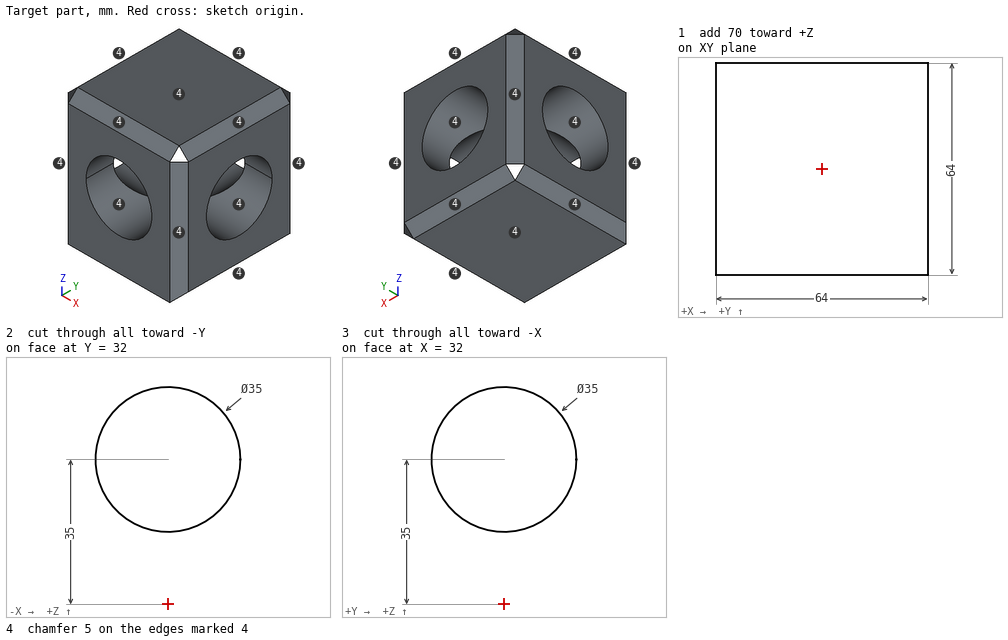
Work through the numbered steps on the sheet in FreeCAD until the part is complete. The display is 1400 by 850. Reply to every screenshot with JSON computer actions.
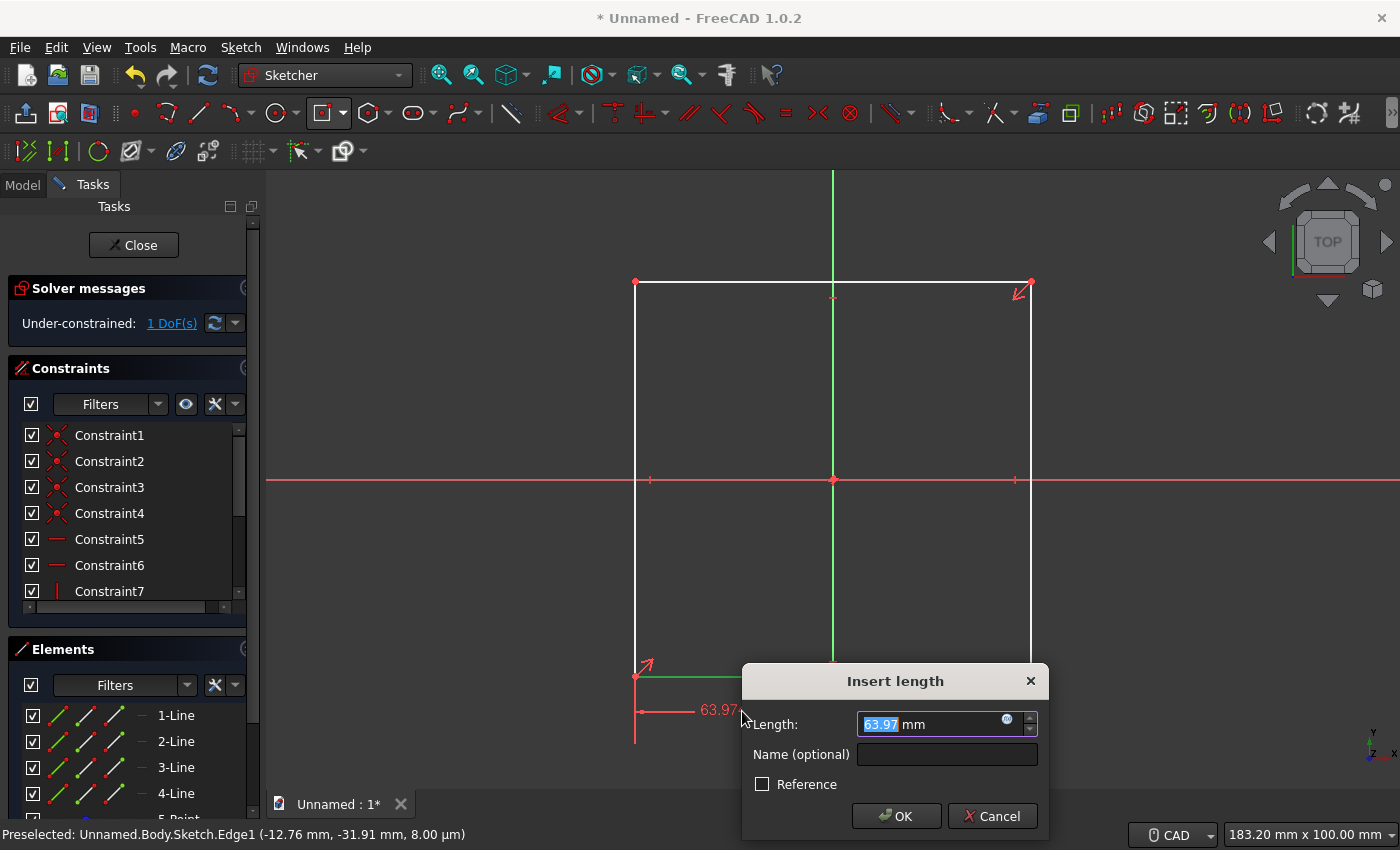
{"action": "type", "text": "64"}
{"action": "key", "text": "Return"}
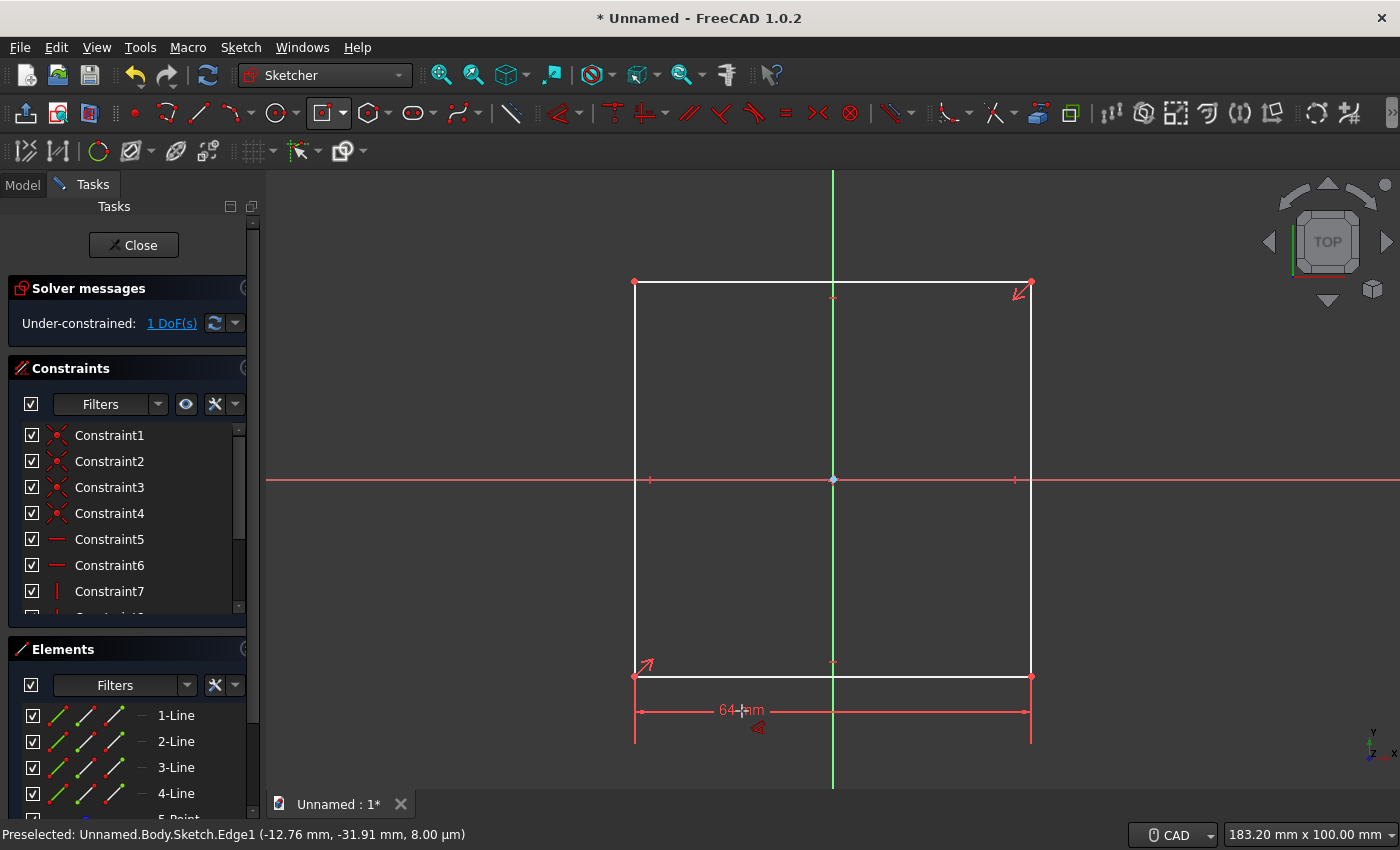
{"action": "left_click", "coordinate": [1031, 559]}
{"action": "left_click", "coordinate": [1065, 389]}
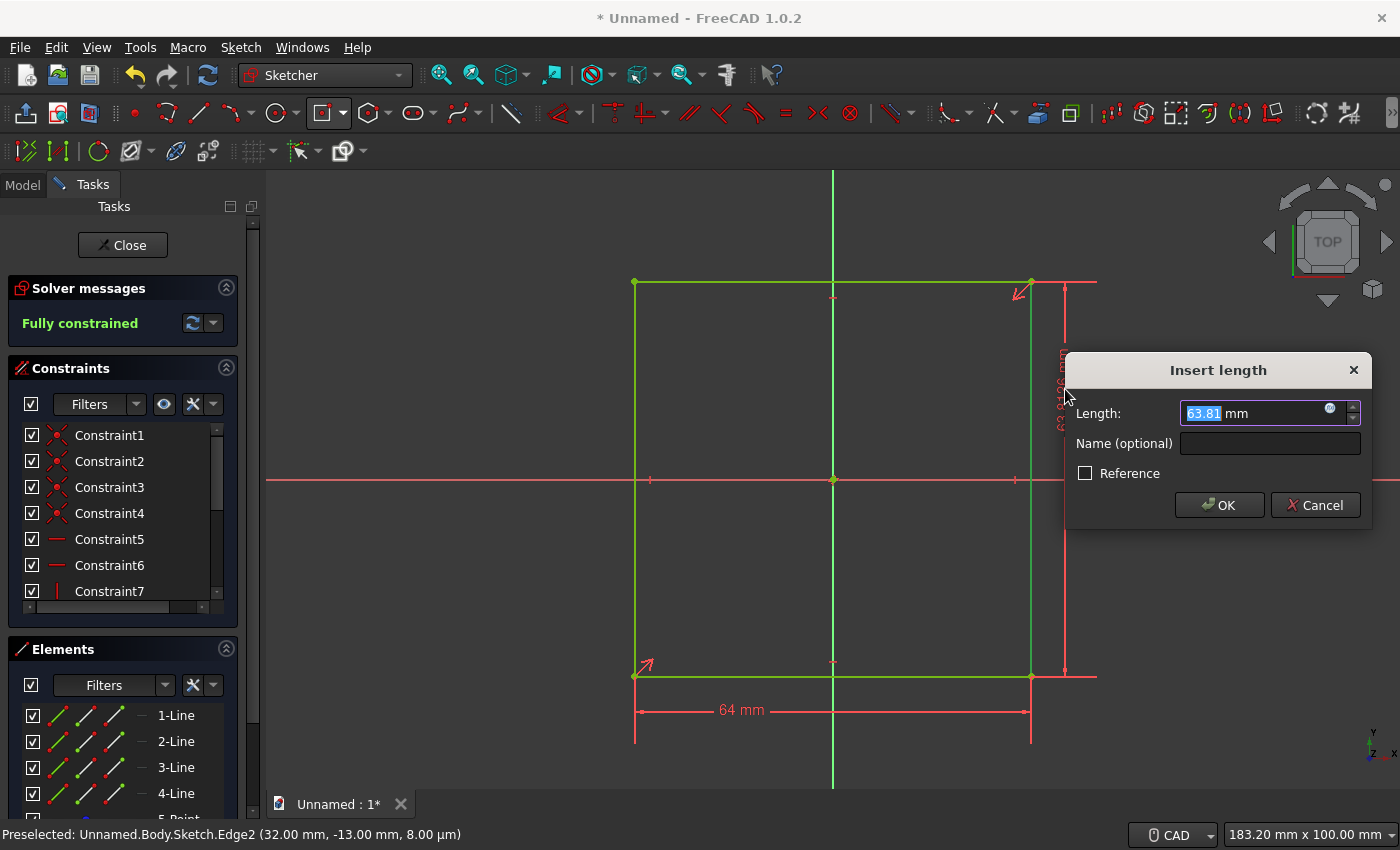
{"action": "type", "text": "64"}
{"action": "key", "text": "Return"}
{"action": "key", "text": "Escape"}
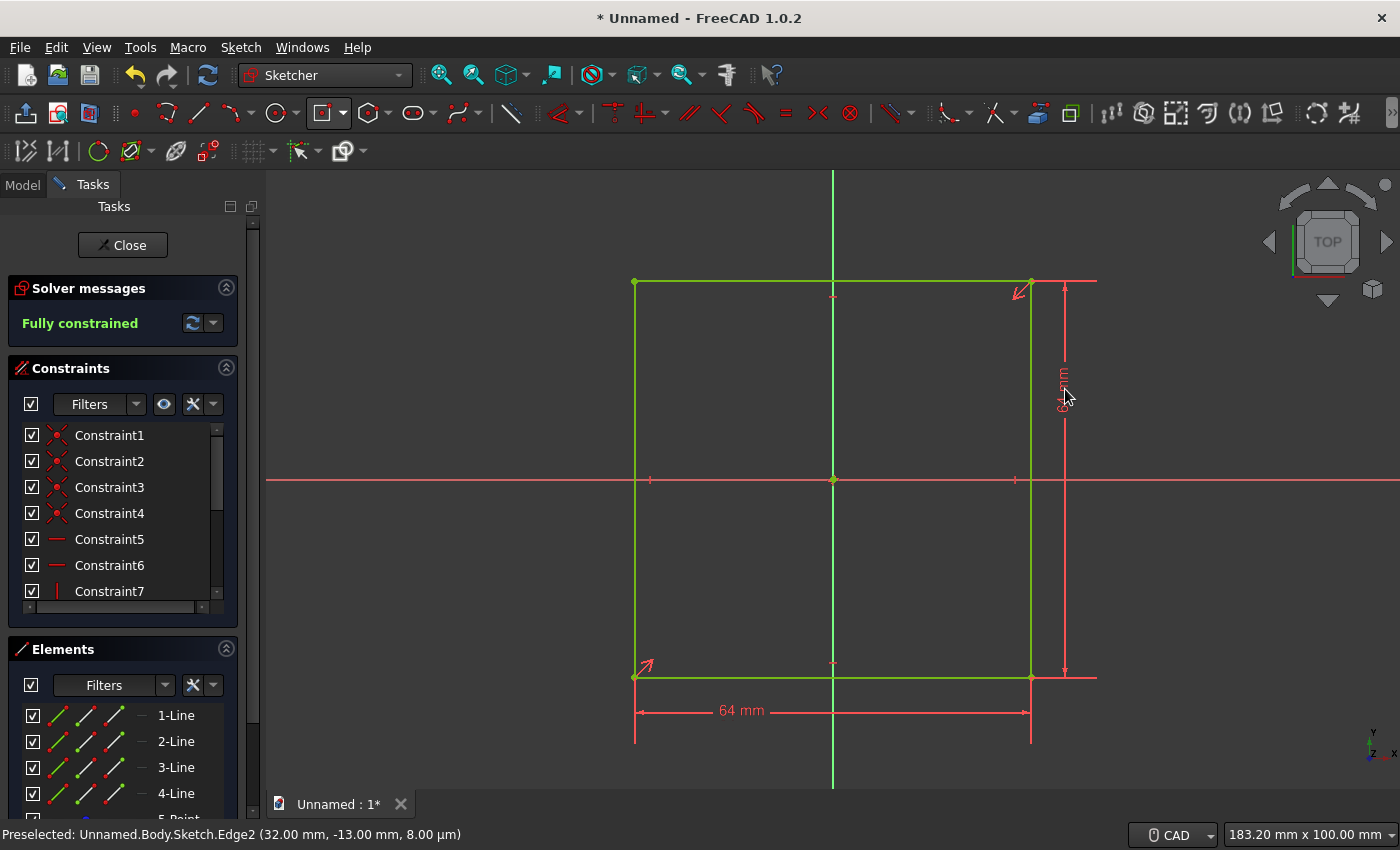
{"action": "left_click", "coordinate": [123, 245]}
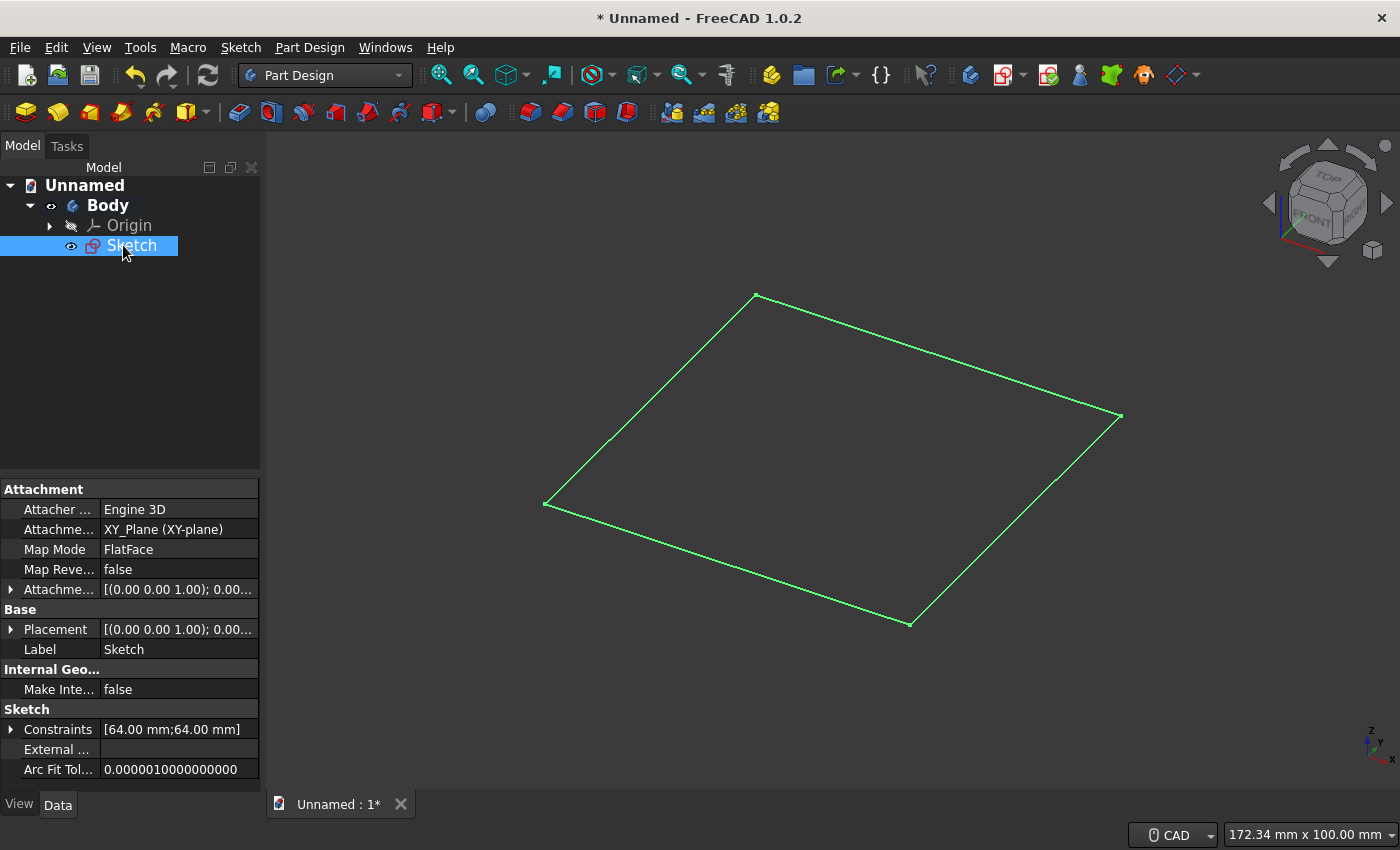
{"action": "left_click", "coordinate": [26, 112]}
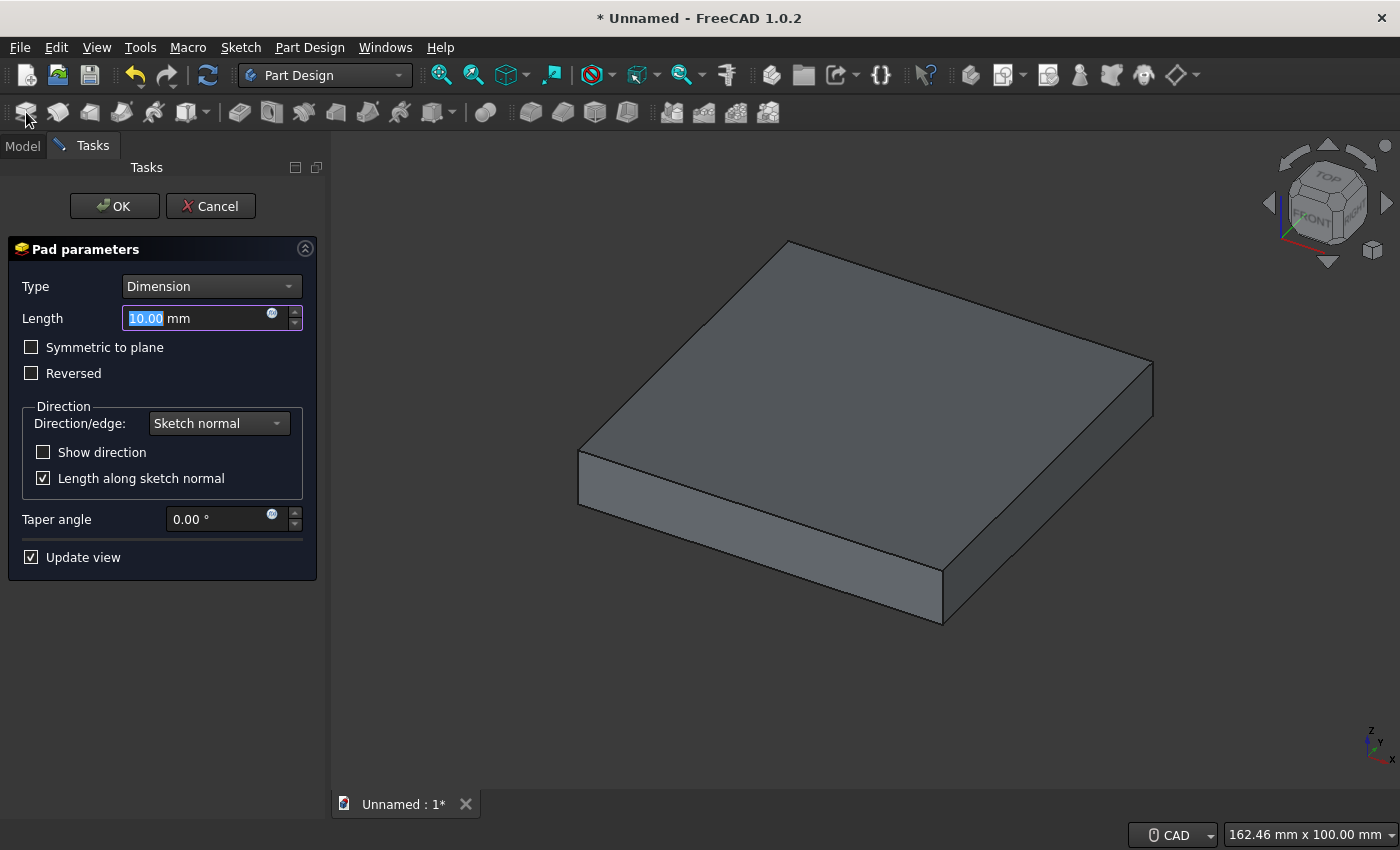
{"action": "type", "text": "70"}
{"action": "key", "text": "Tab"}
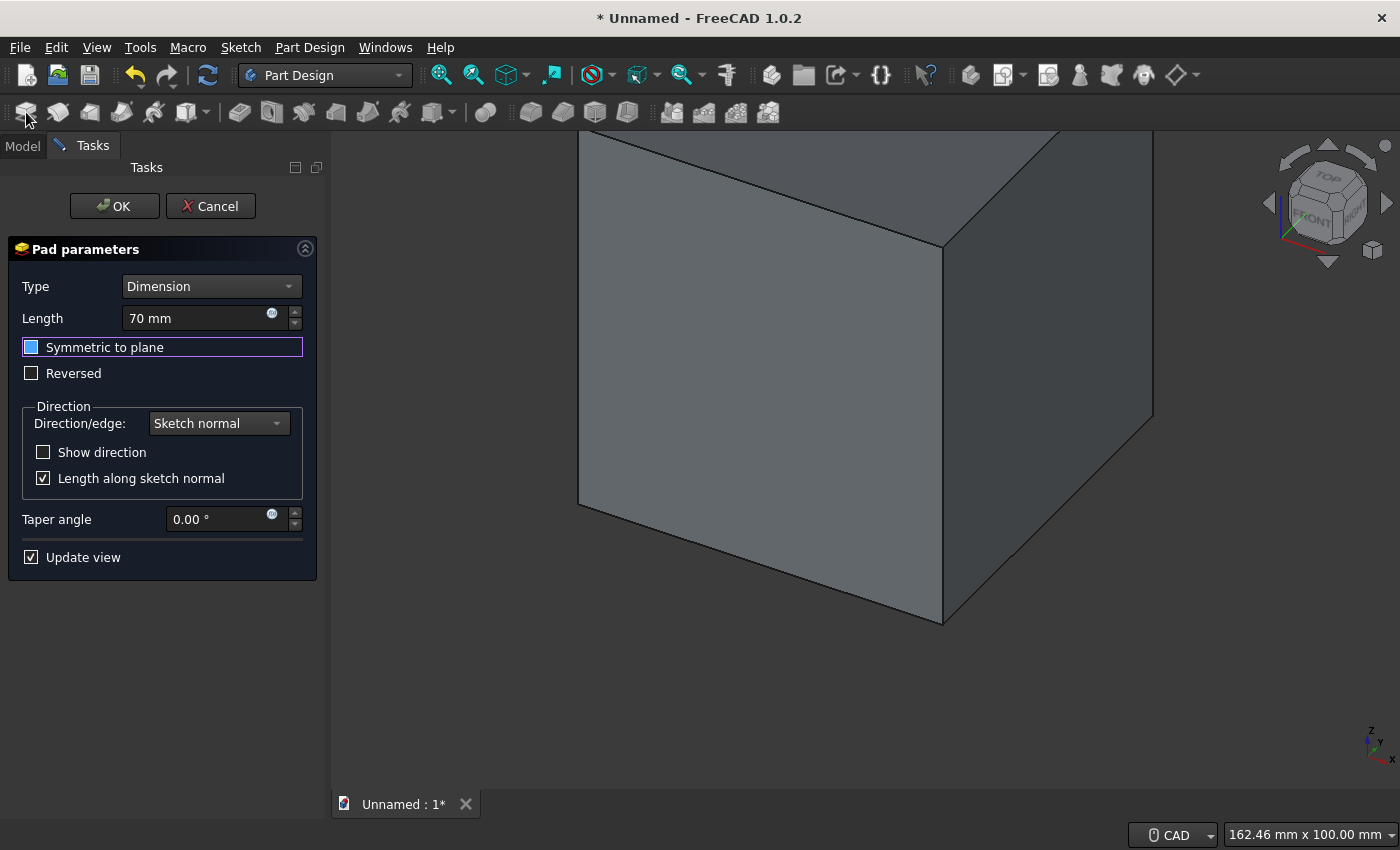
{"action": "left_click", "coordinate": [115, 206]}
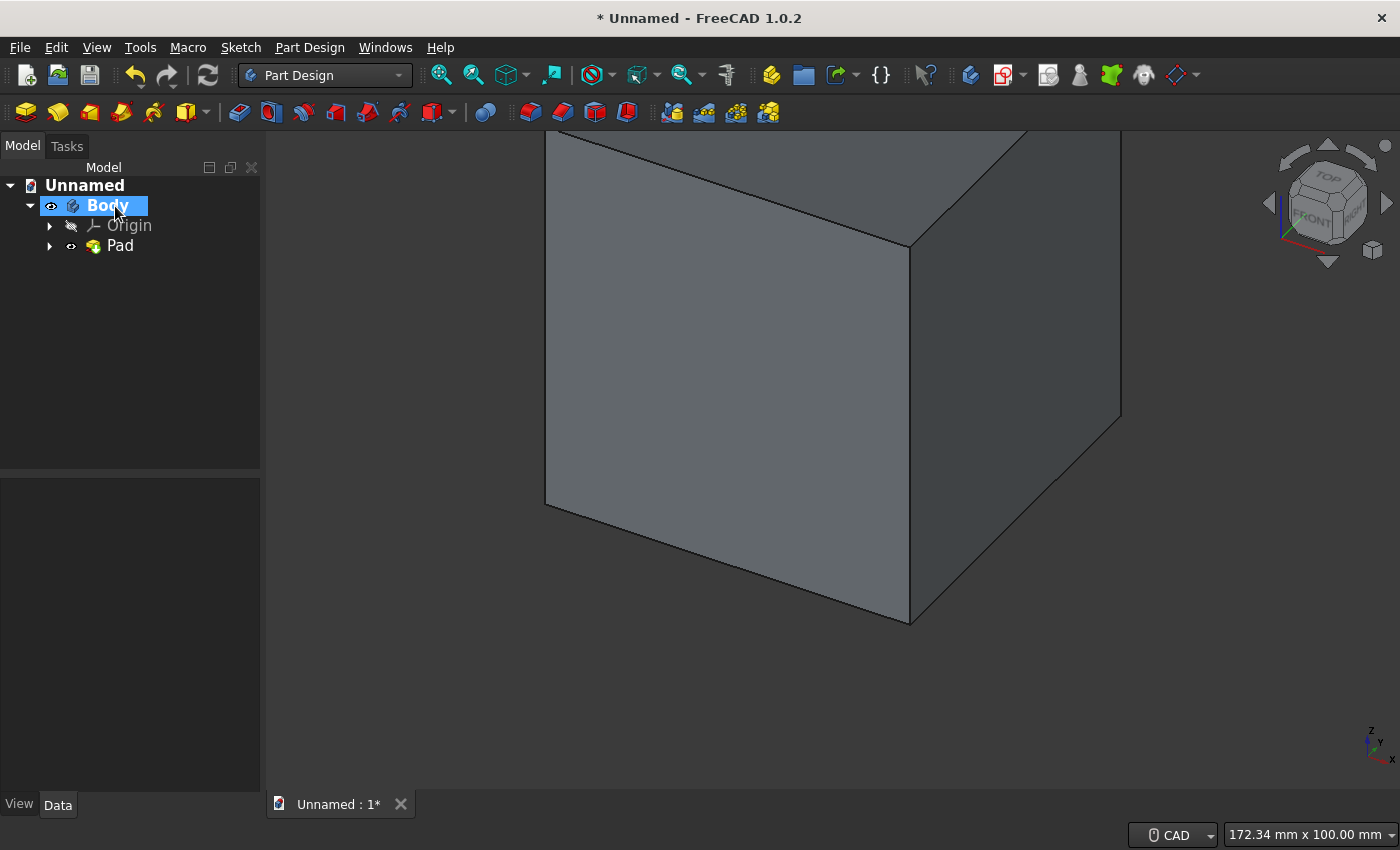
{"action": "key", "text": "v f"}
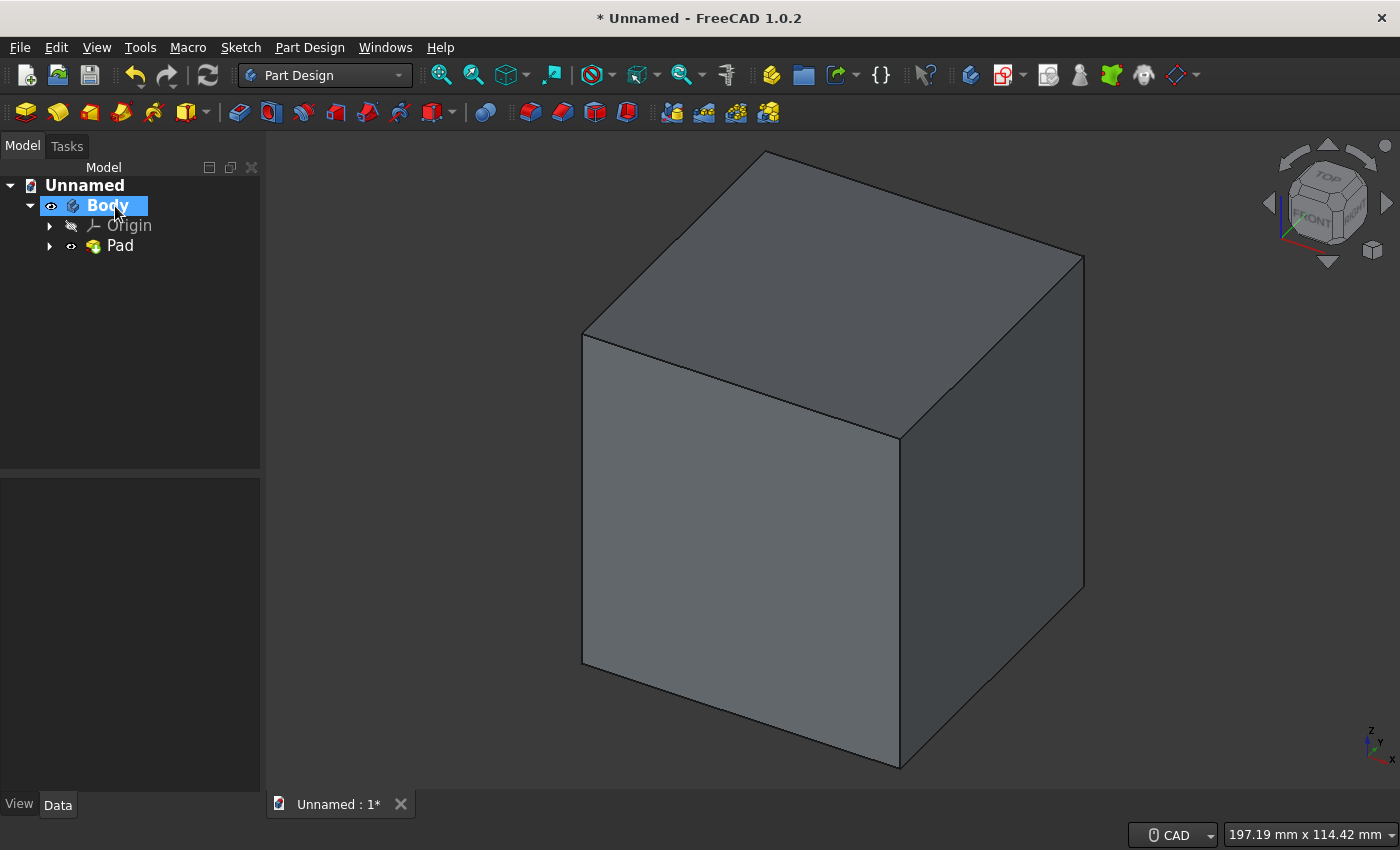
{"action": "key", "text": "4"}